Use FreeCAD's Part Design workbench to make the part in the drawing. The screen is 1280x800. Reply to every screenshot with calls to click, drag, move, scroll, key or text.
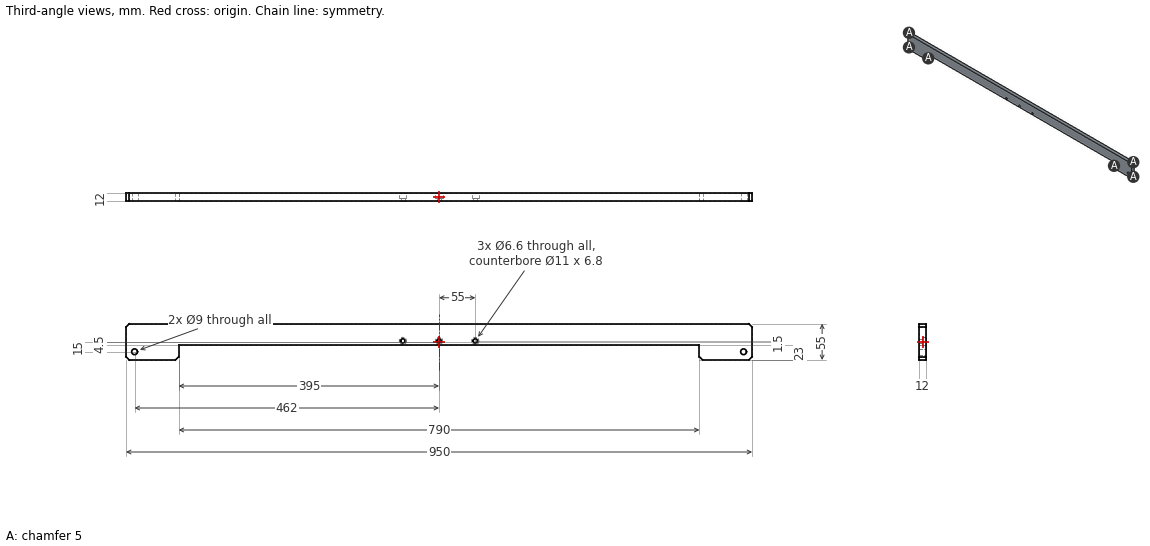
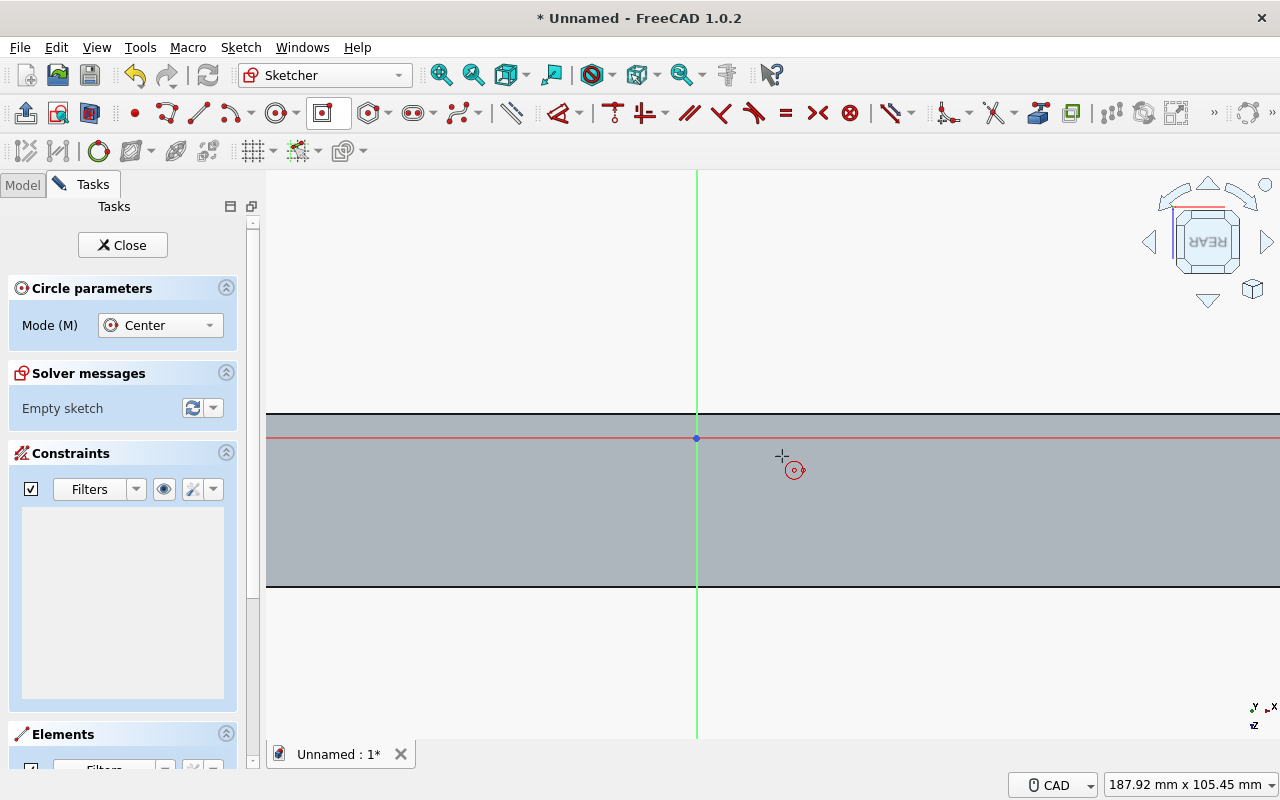
scroll(993, 447, up, 4)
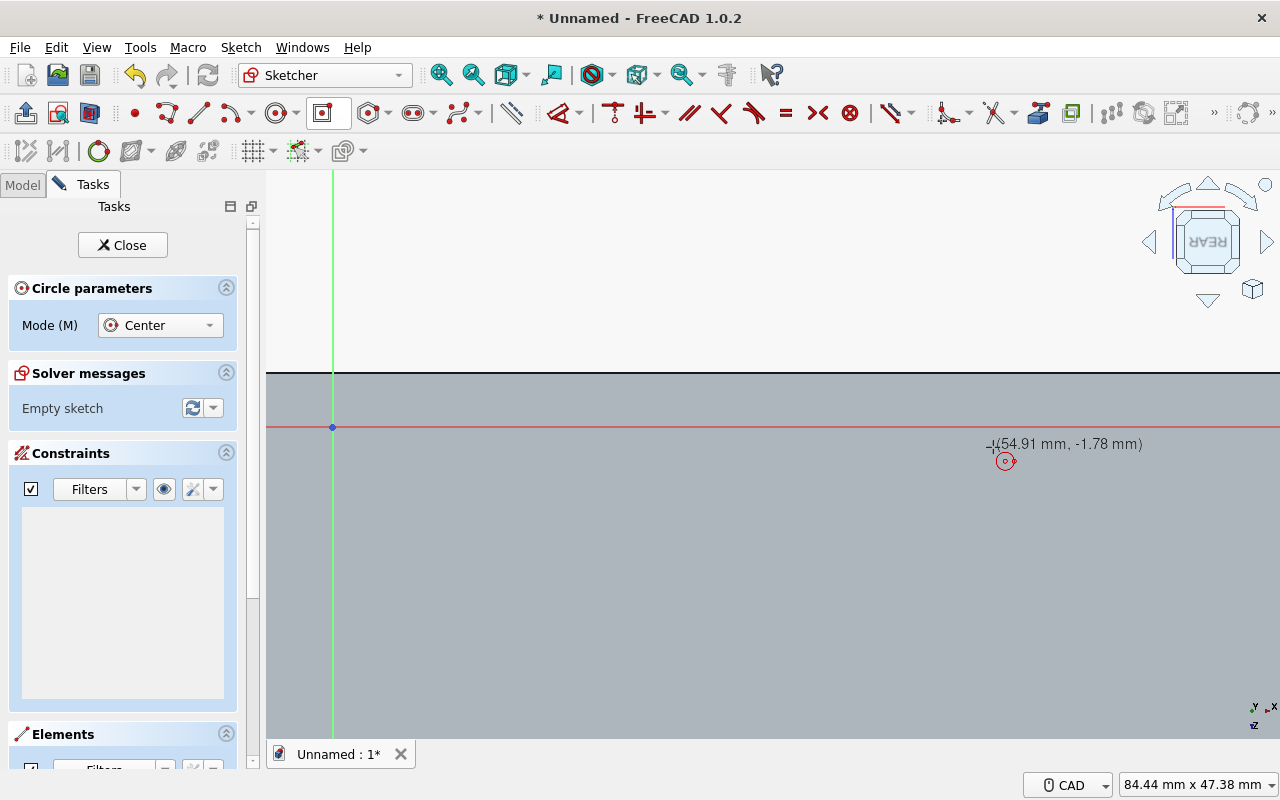
click(993, 445)
move(1021, 473)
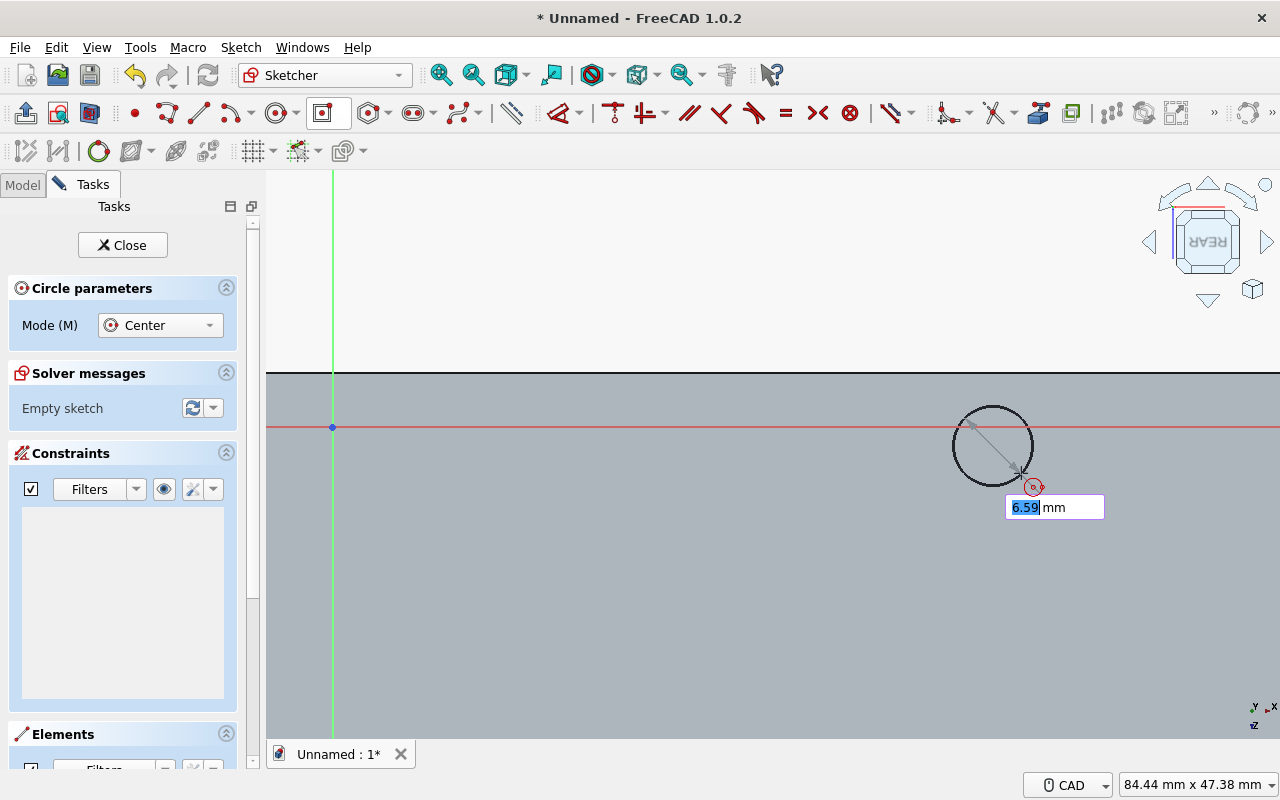
text(6.6)
key(Return)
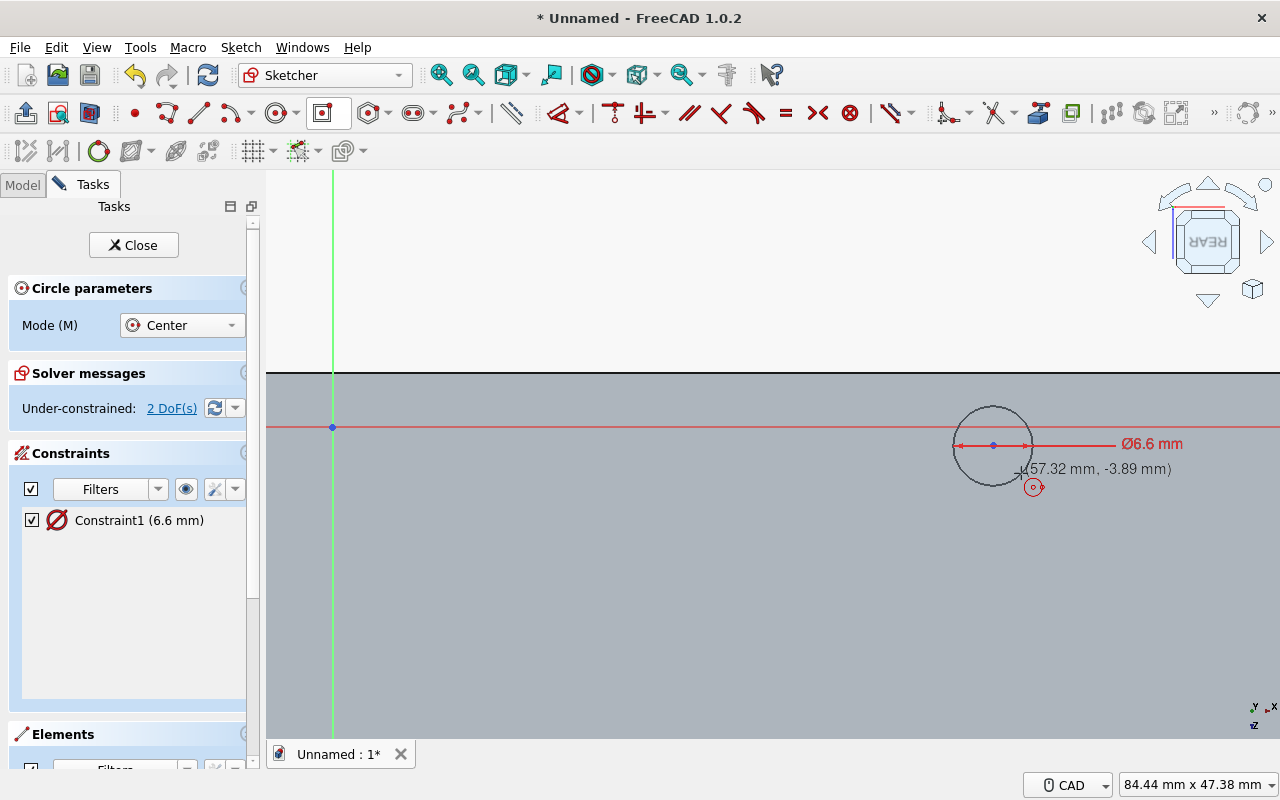
click(333, 445)
move(361, 473)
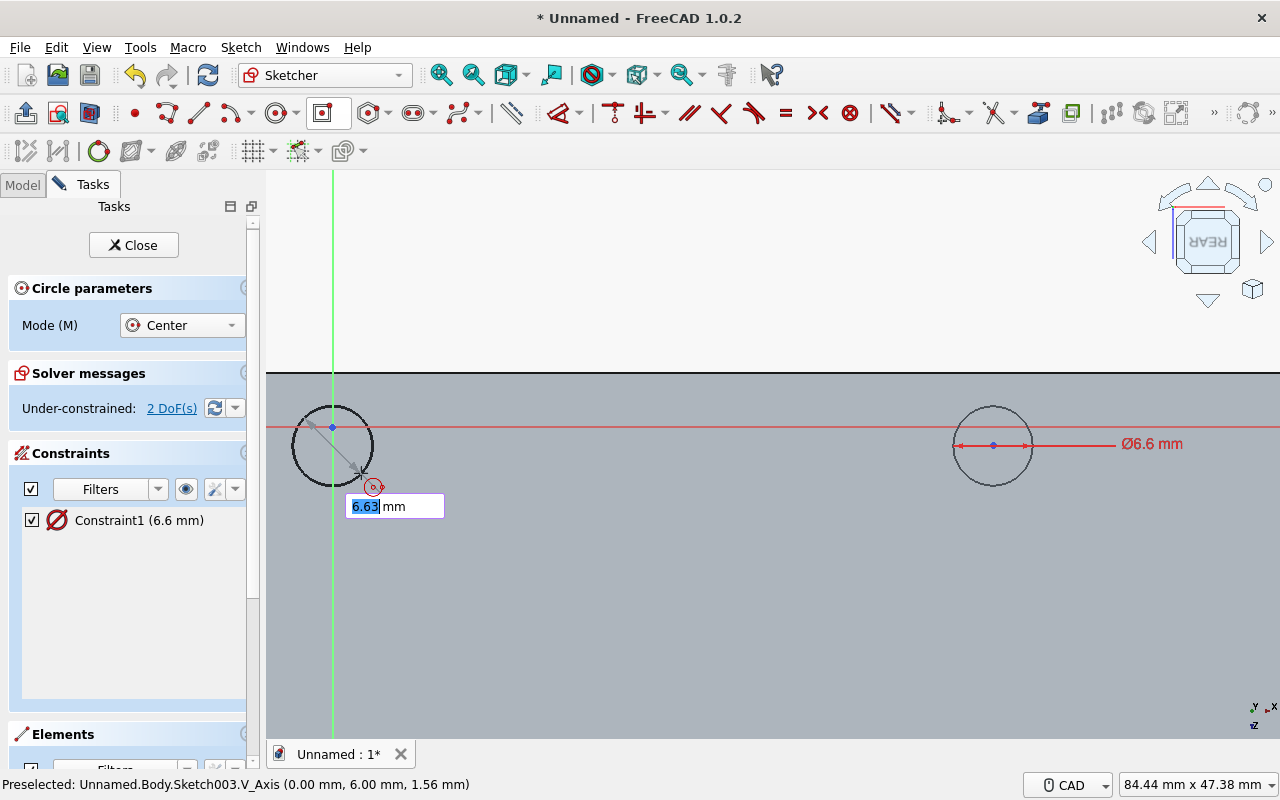
text(6.6)
key(Return)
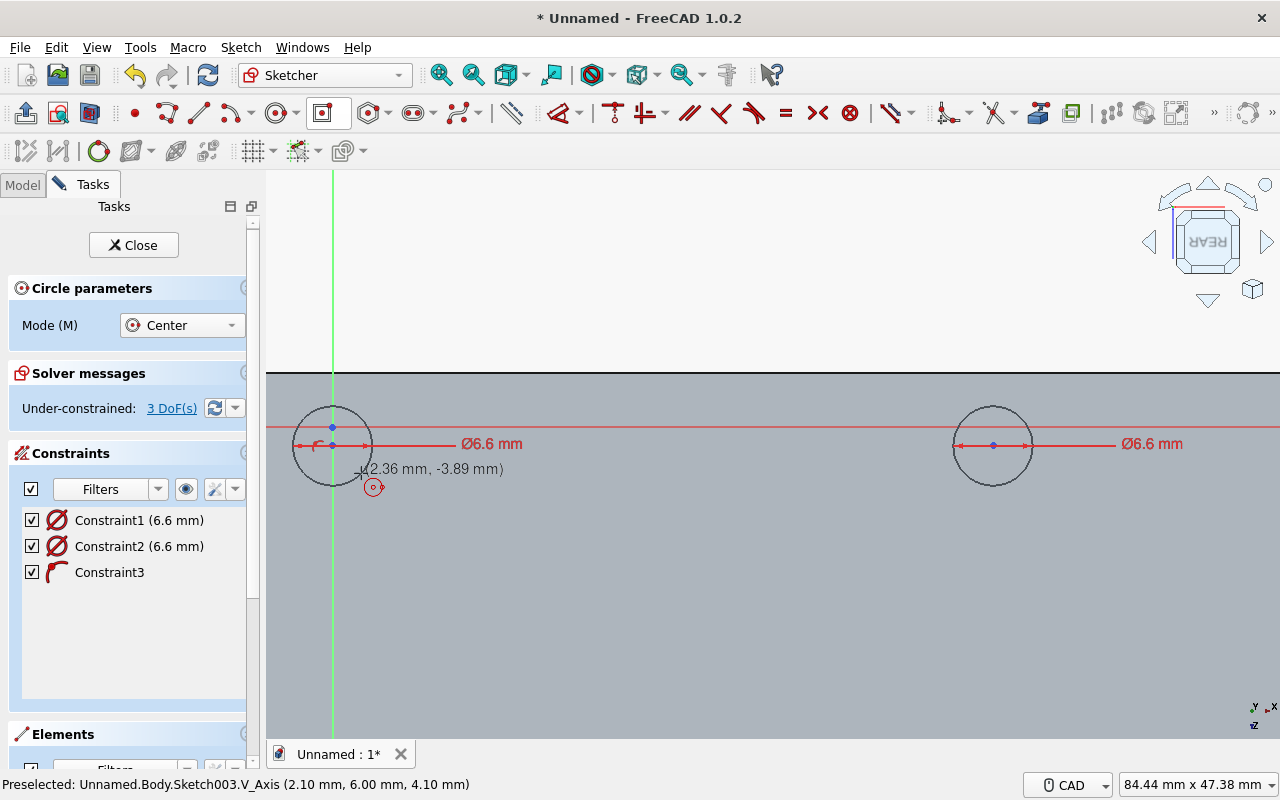
scroll(1008, 462, down, 4)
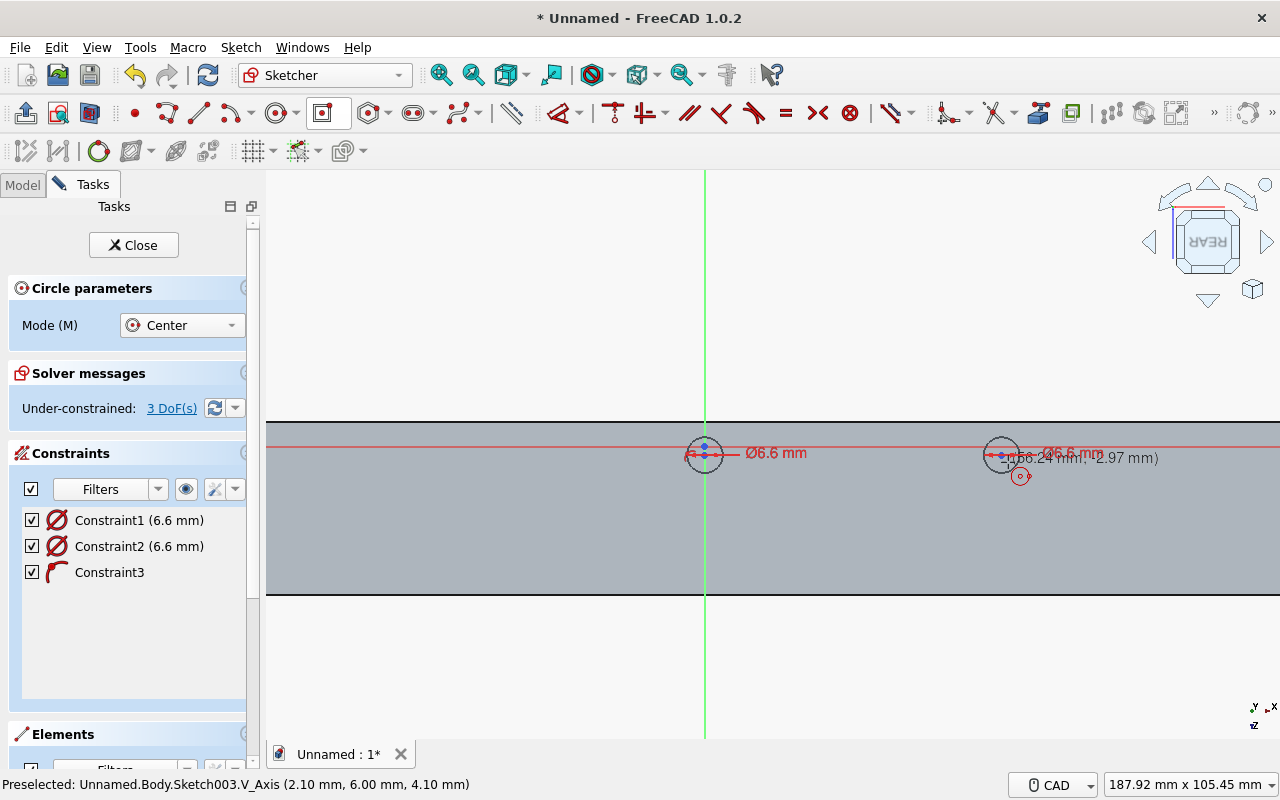
scroll(408, 455, up, 4)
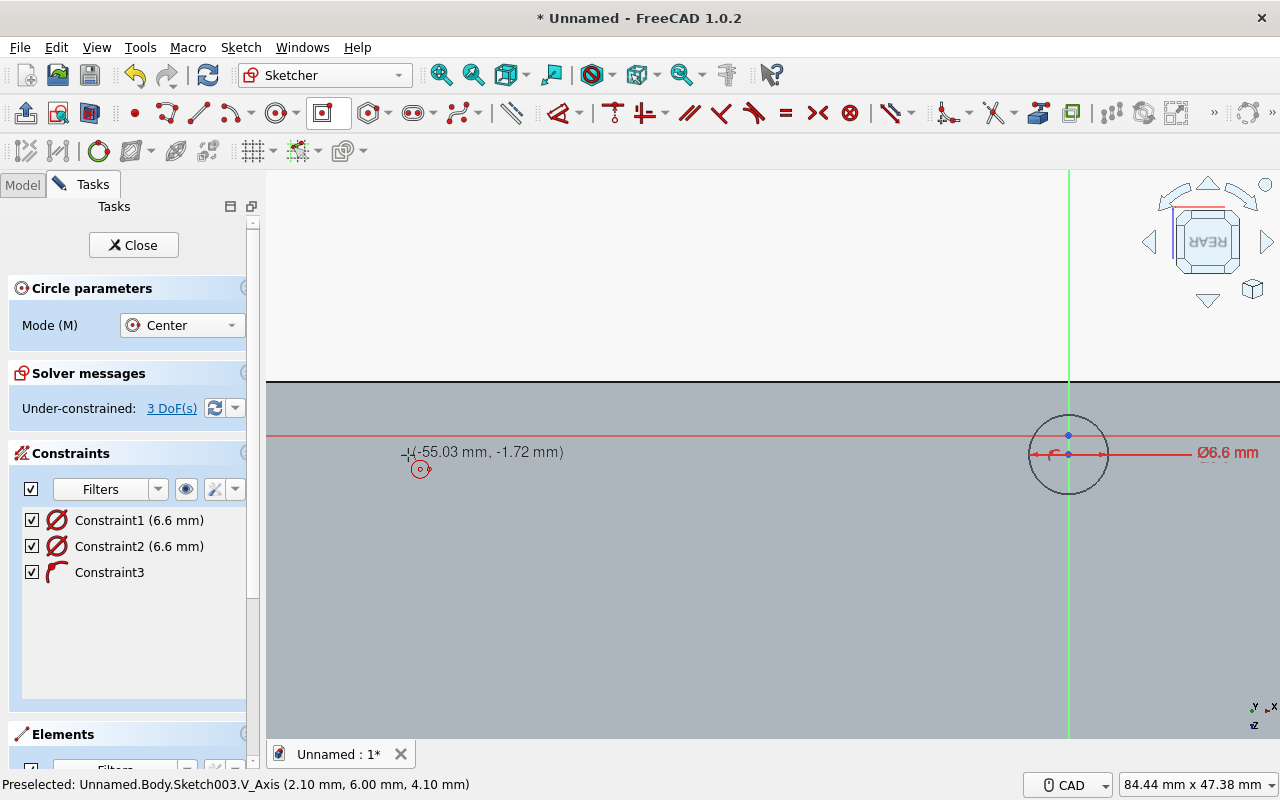
click(408, 454)
move(436, 482)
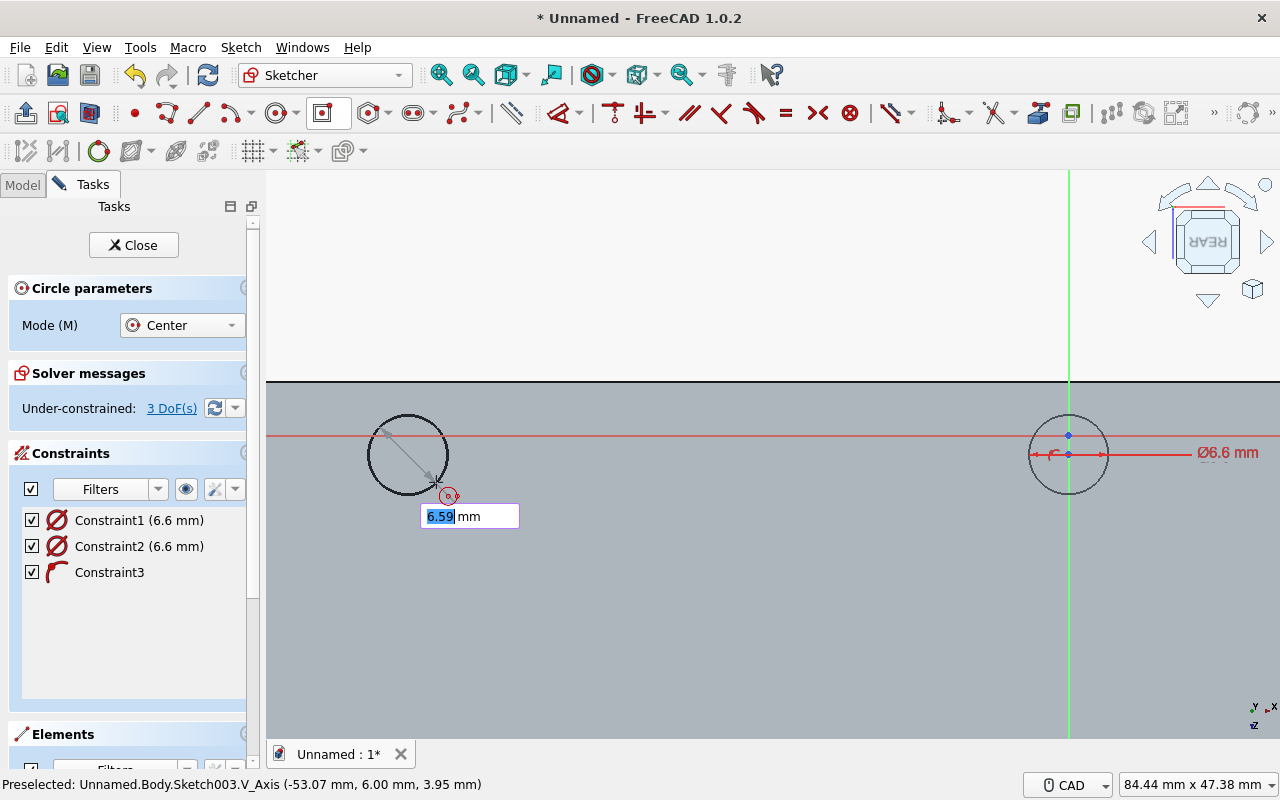
text(6.6)
key(Return)
key(Escape)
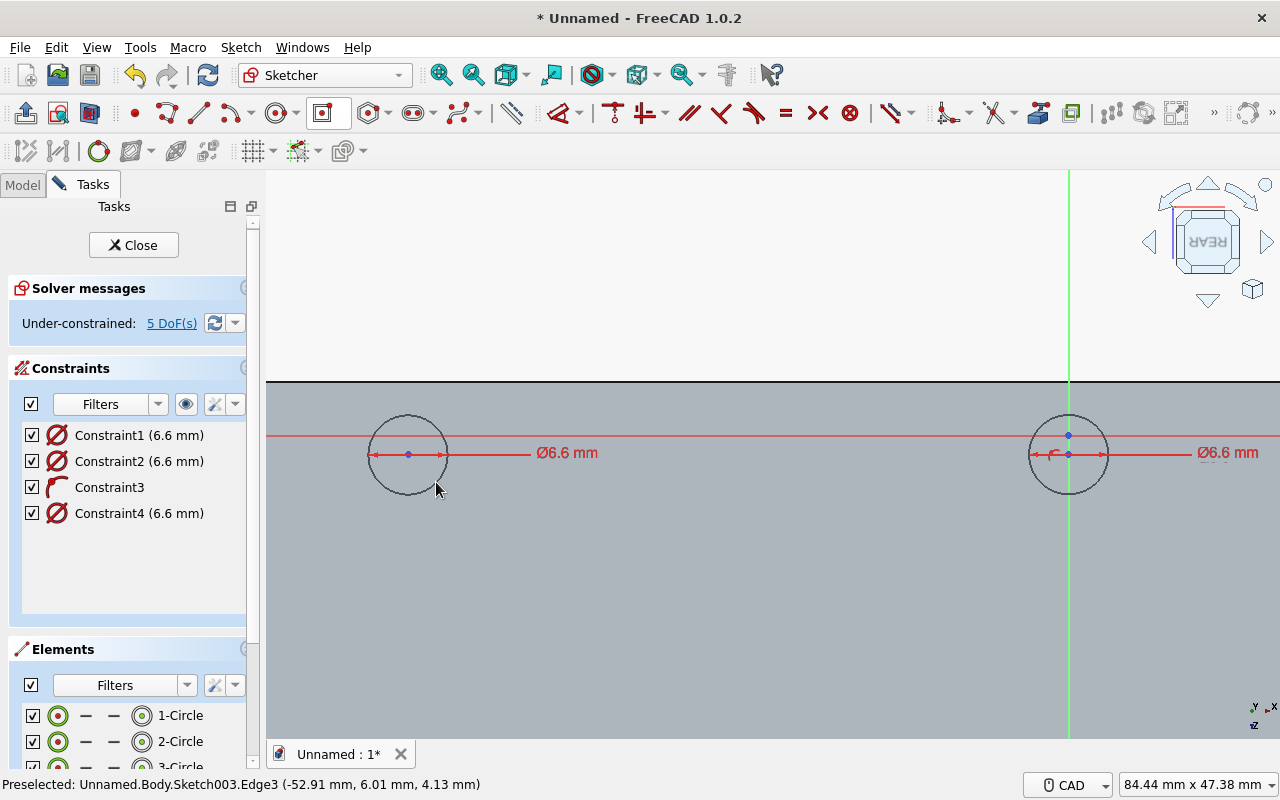
scroll(407, 455, down, 4)